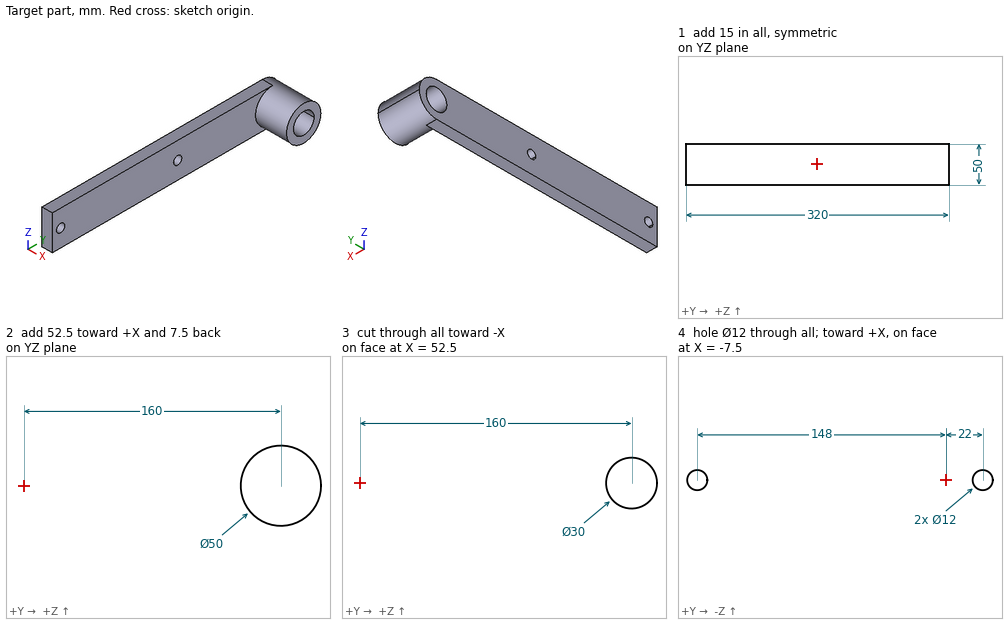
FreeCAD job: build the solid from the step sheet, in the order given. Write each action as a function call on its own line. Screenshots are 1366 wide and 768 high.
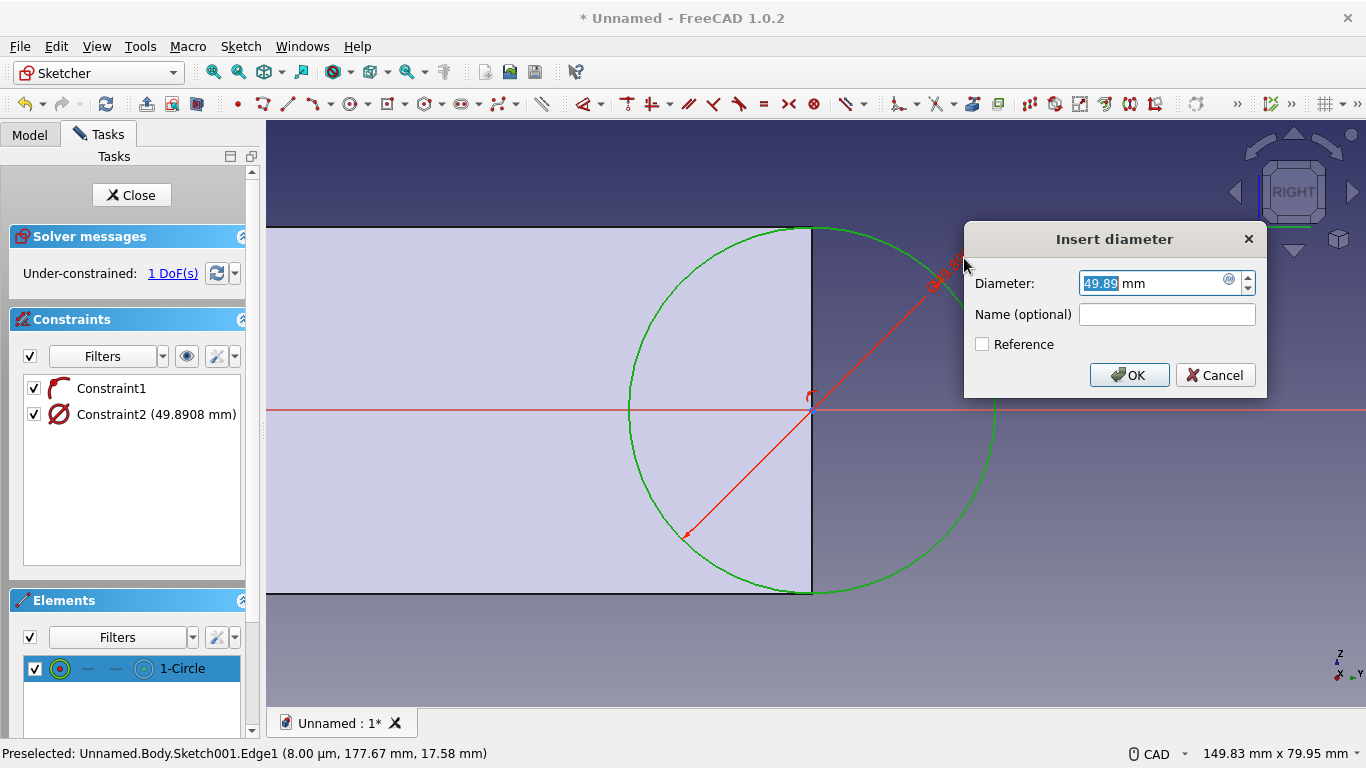
text(50)
key(Return)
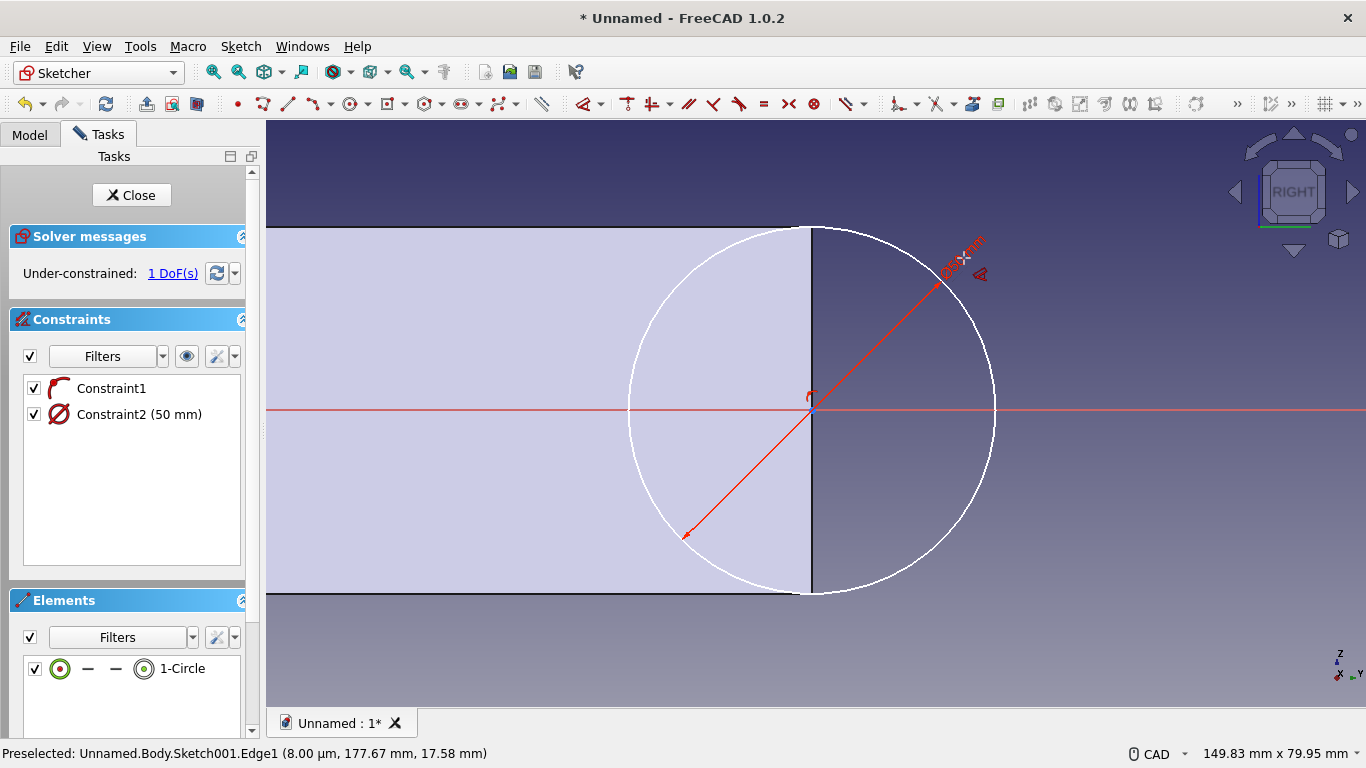
click(812, 410)
click(553, 444)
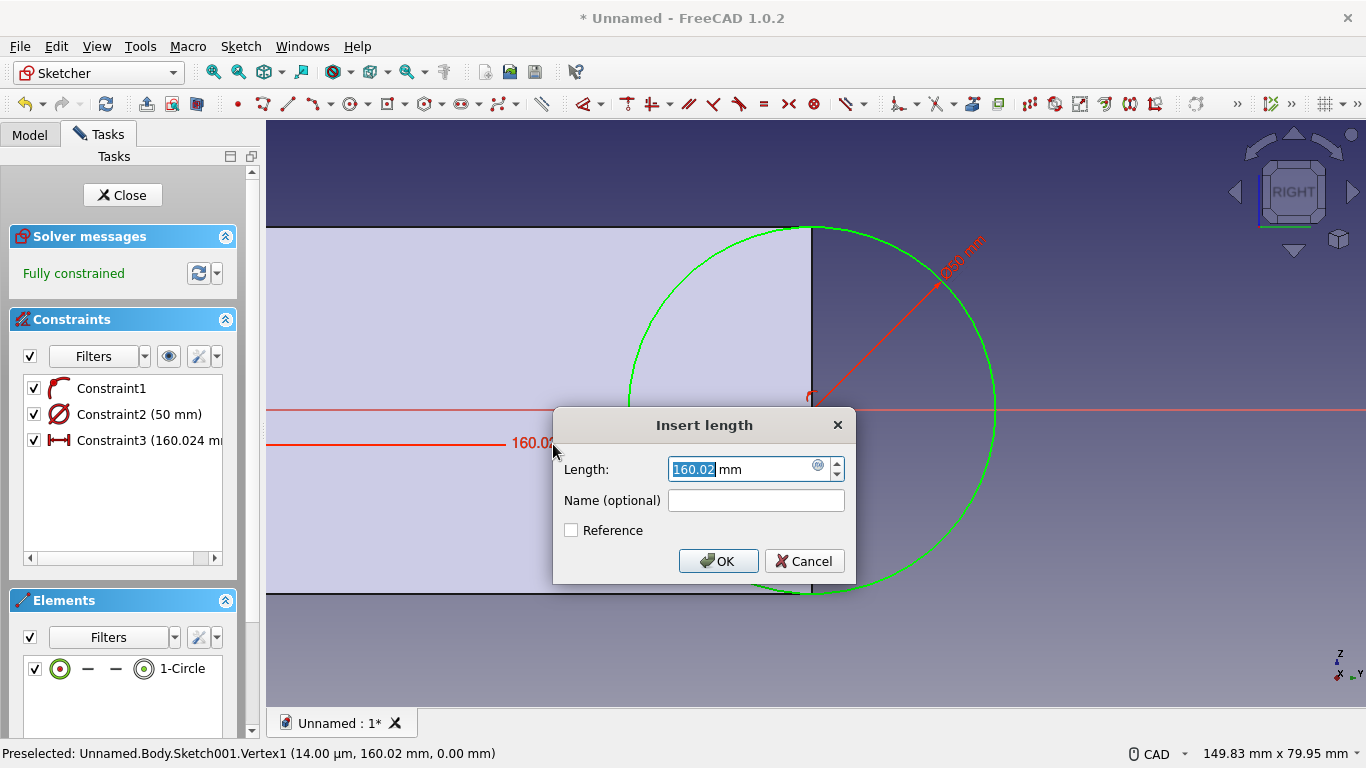
text(160)
key(Return)
key(Escape)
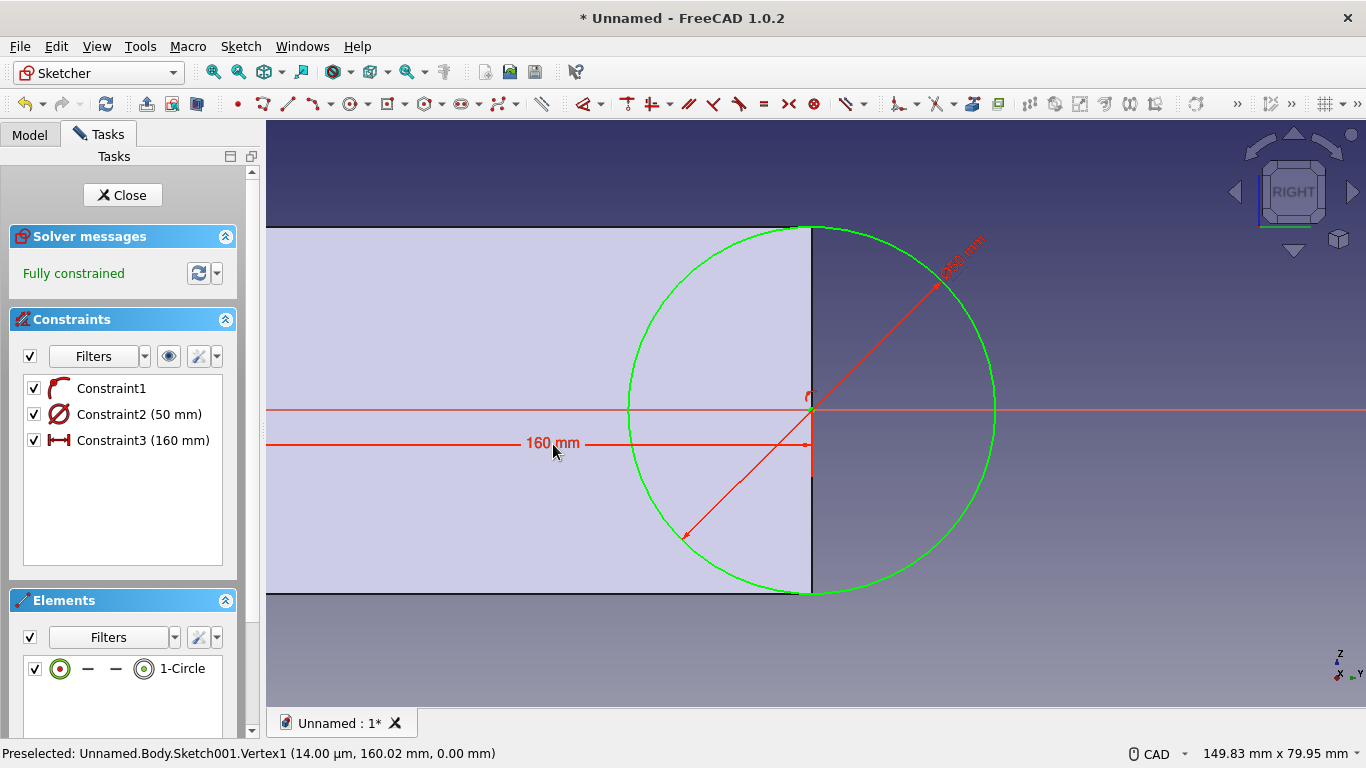
click(123, 195)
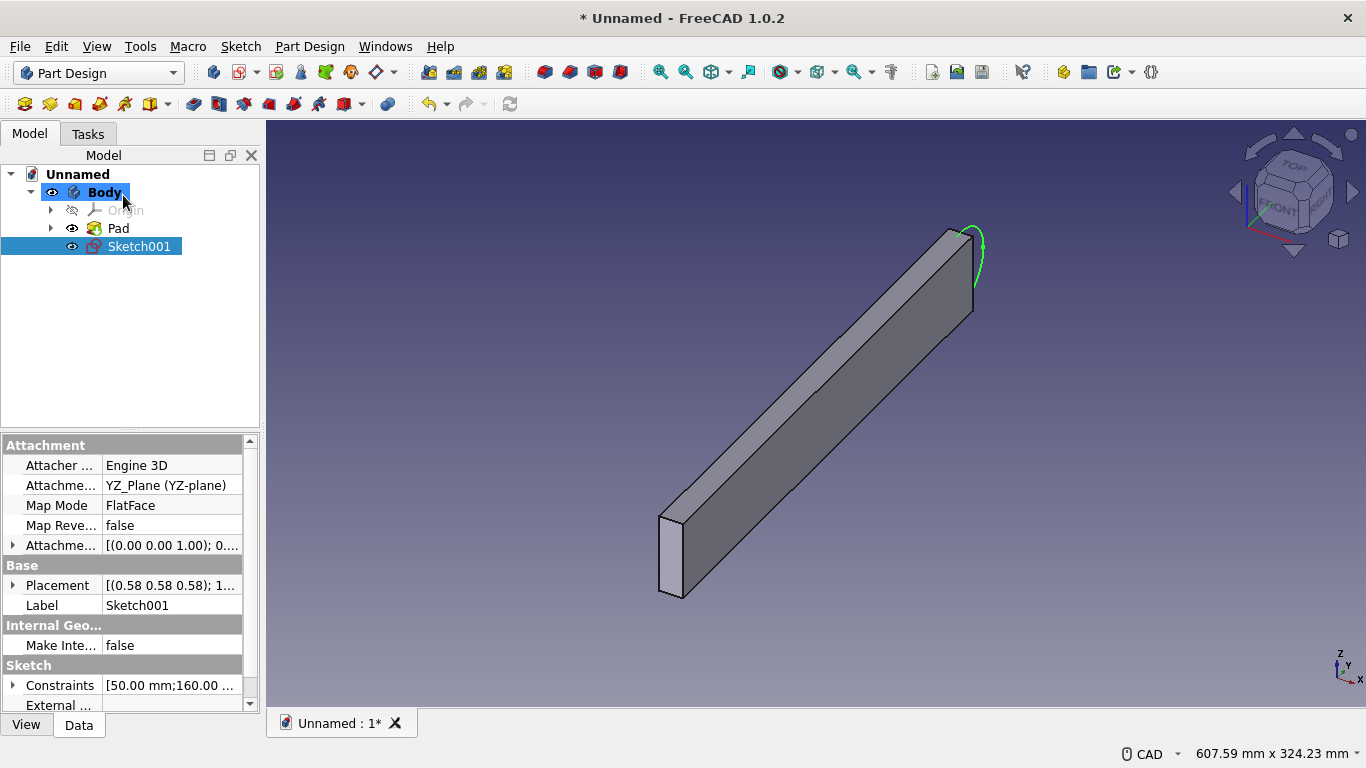
click(25, 104)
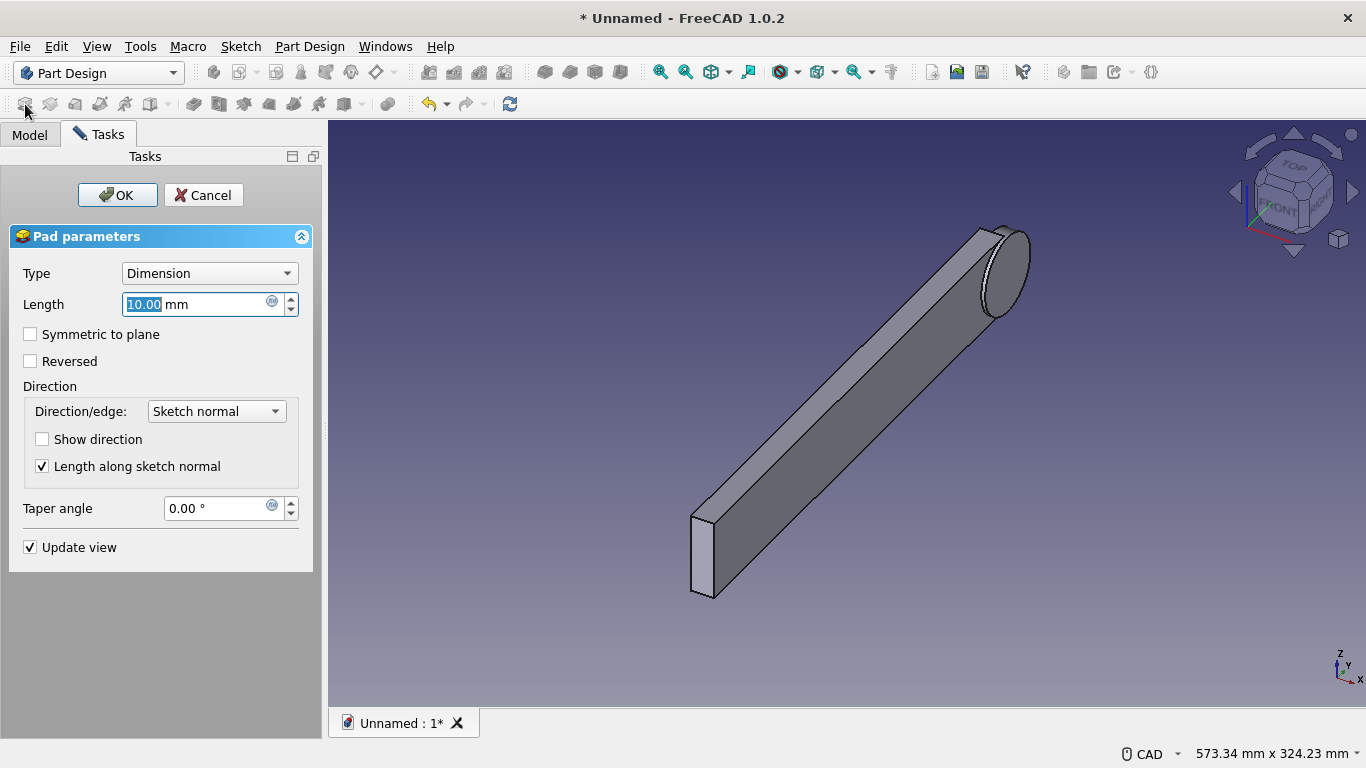
click(210, 274)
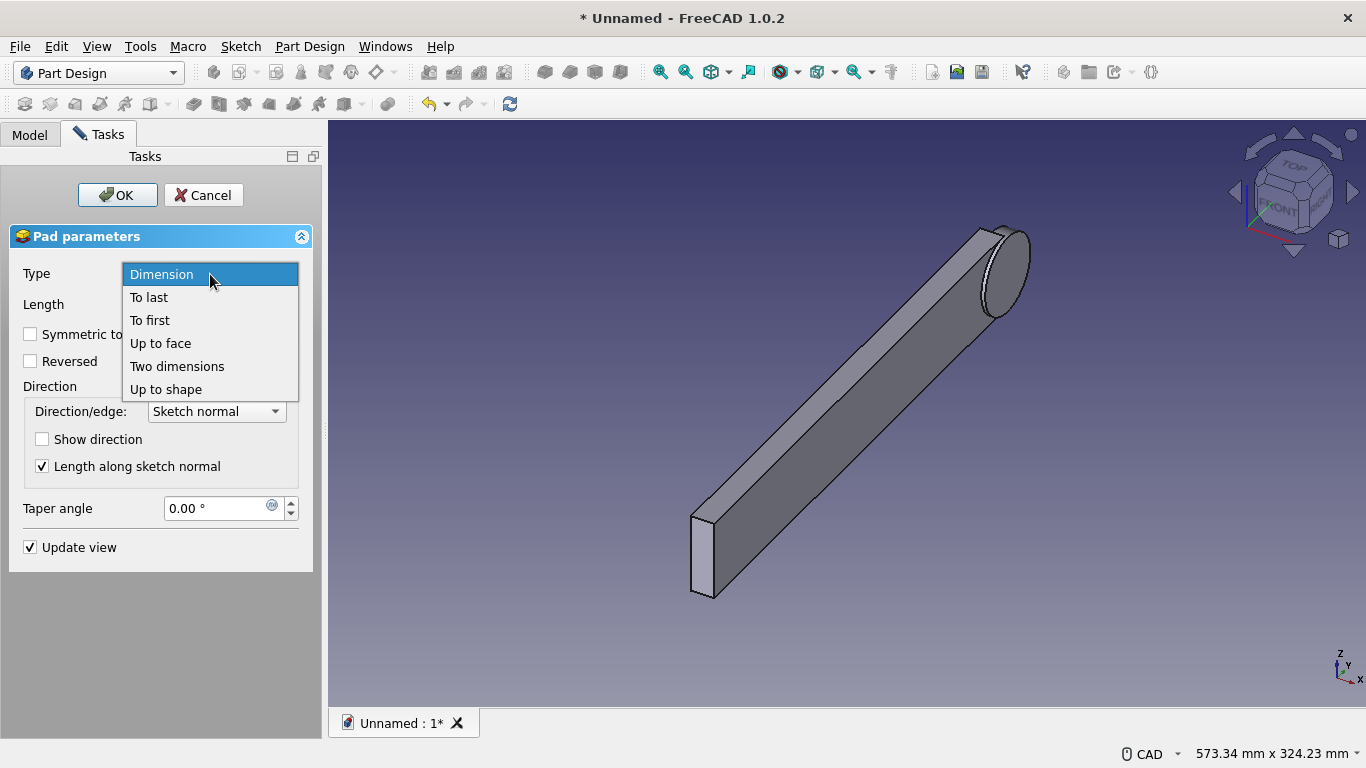
click(208, 366)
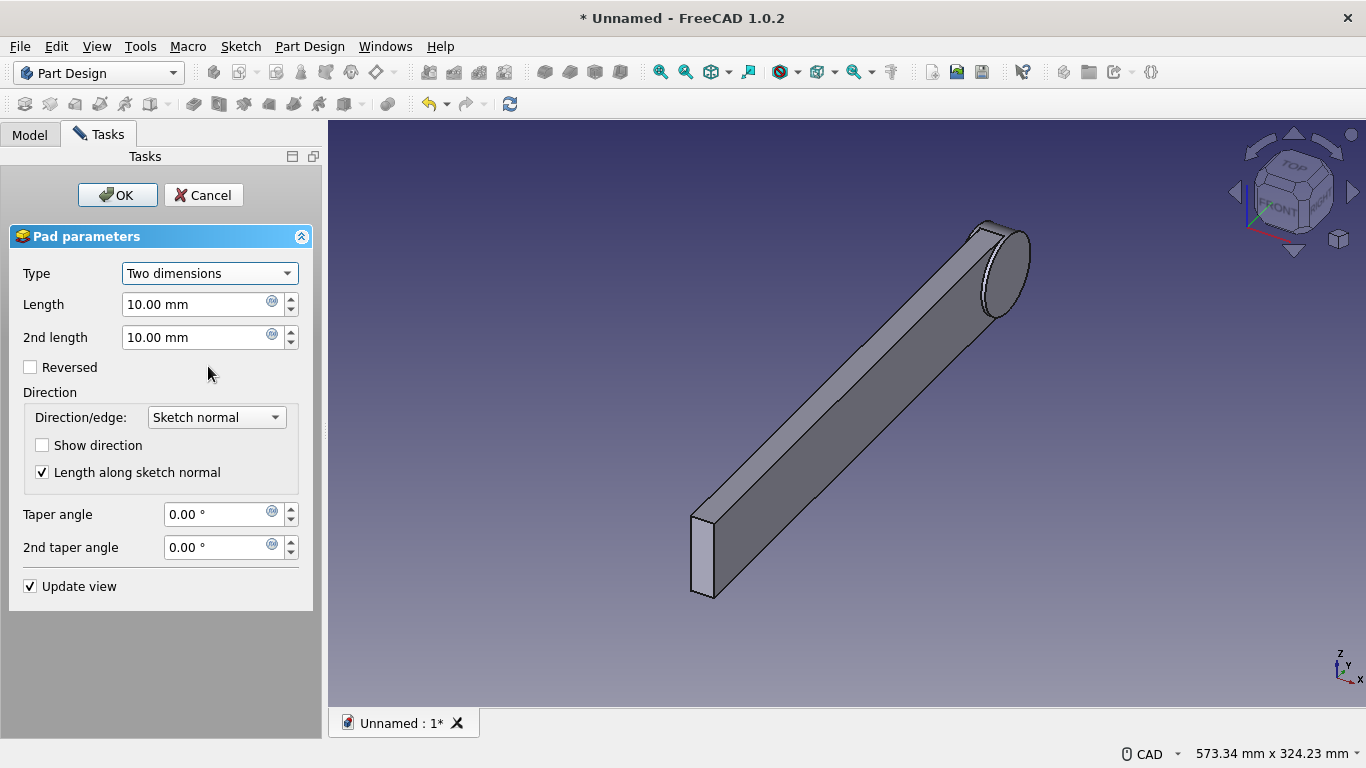
triple_click(204, 304)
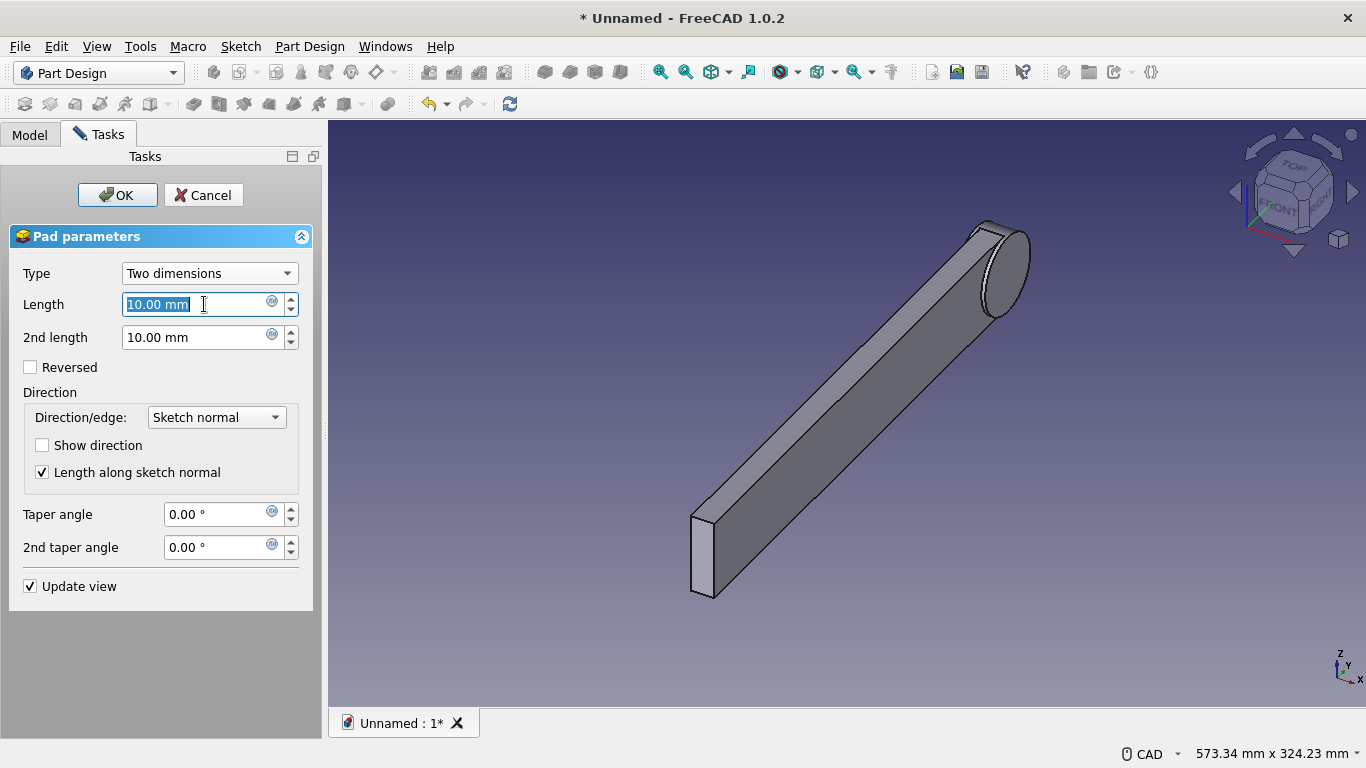
text(52.5)
key(Tab)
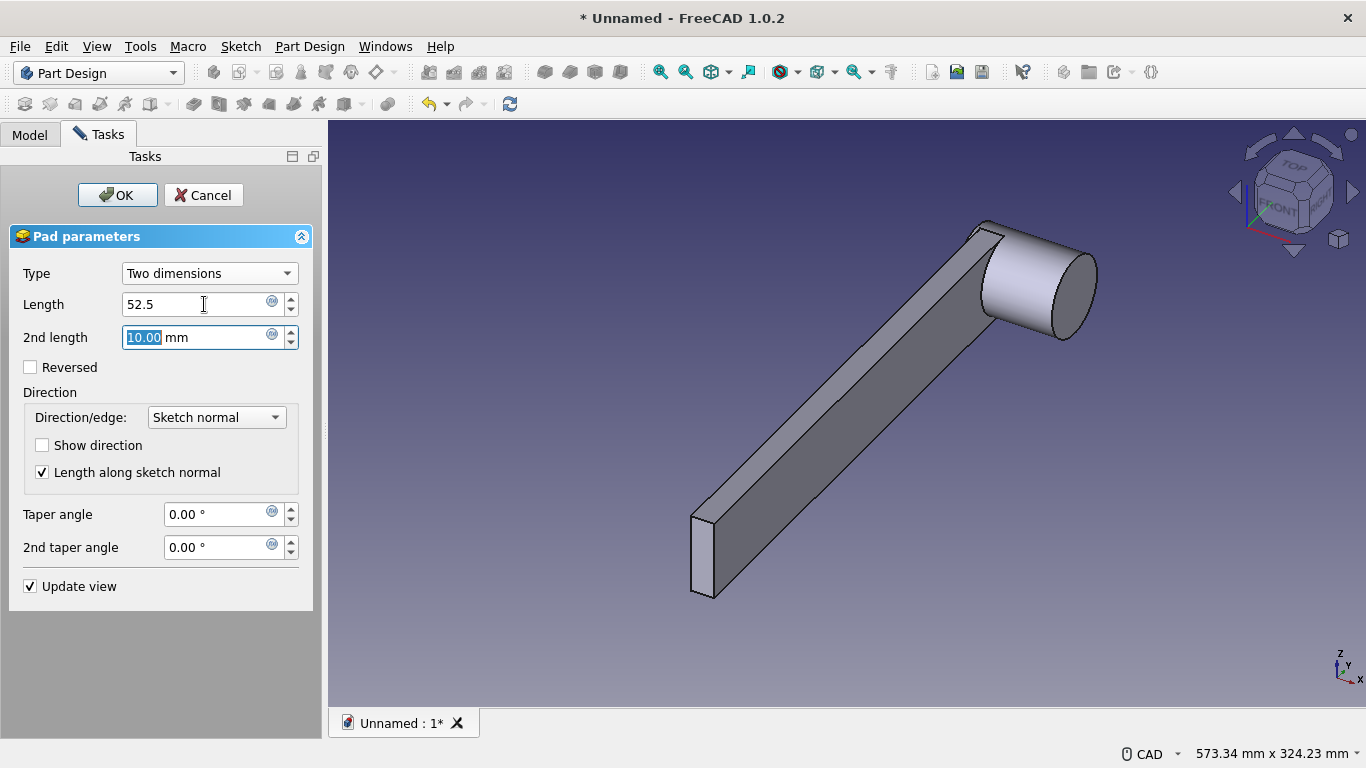
text(7.5)
key(Tab)